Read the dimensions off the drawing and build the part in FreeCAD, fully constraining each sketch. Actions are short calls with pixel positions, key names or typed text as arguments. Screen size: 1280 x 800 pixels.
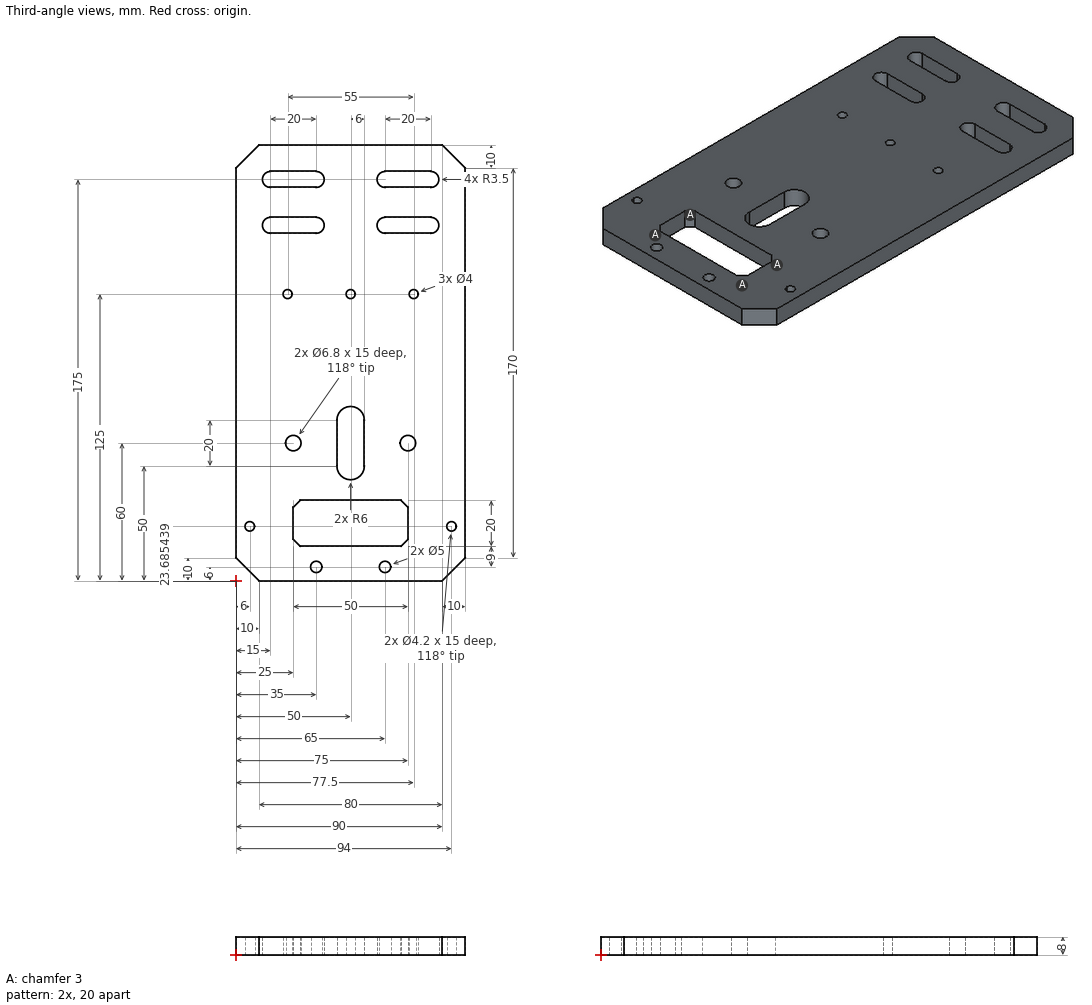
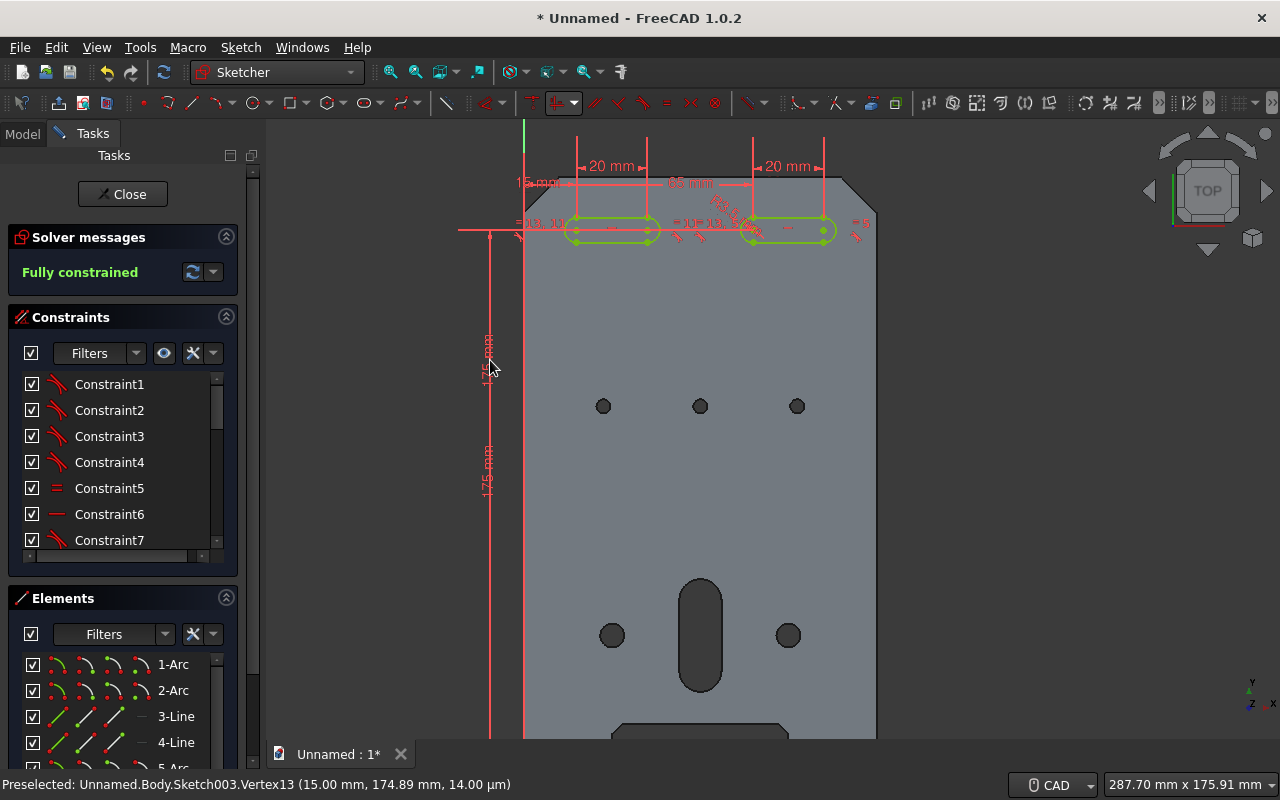
click(123, 194)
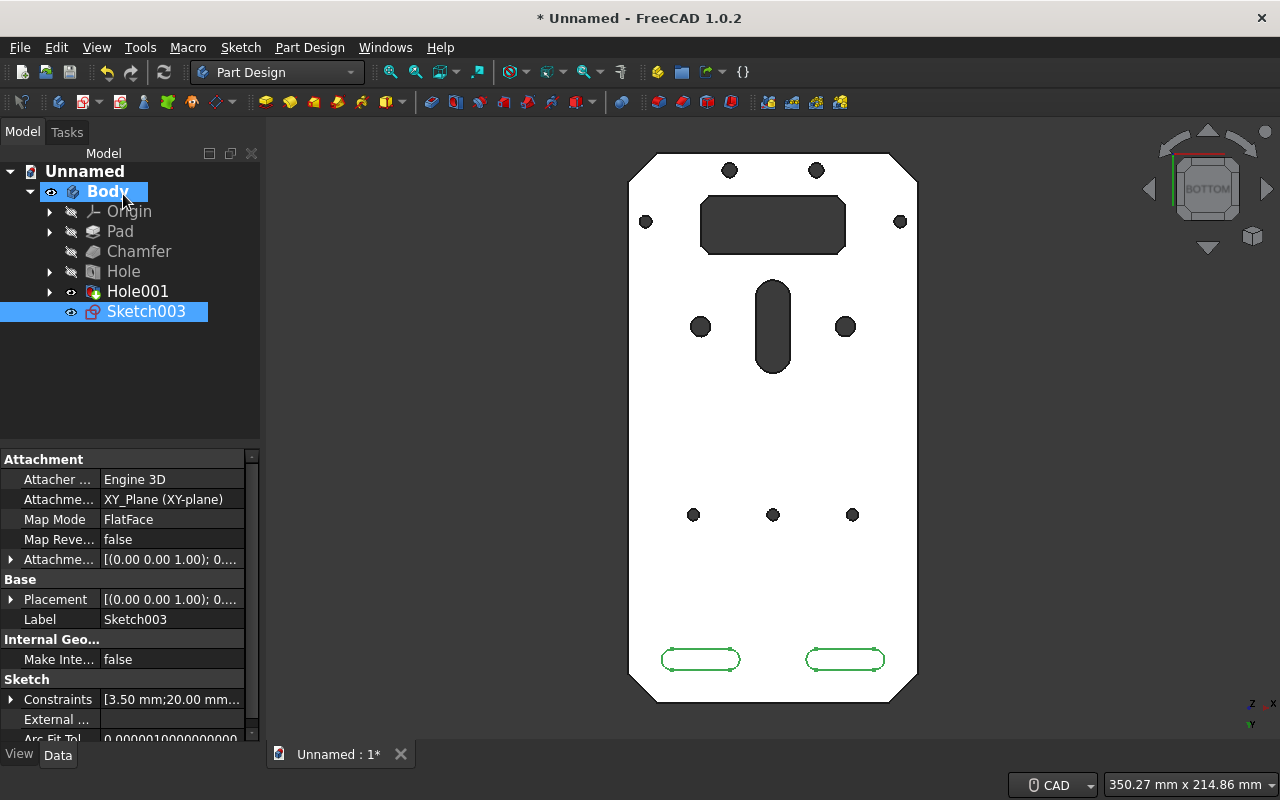
click(432, 102)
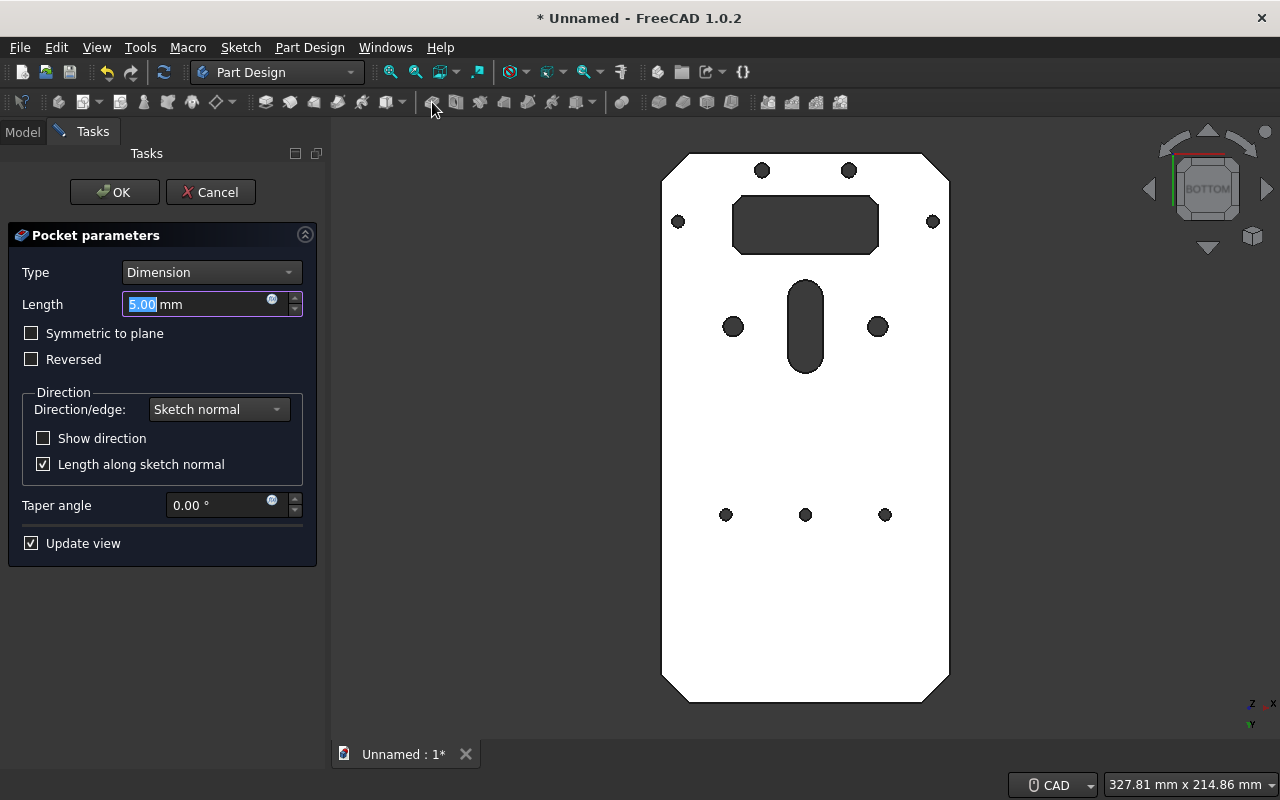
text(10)
key(Tab)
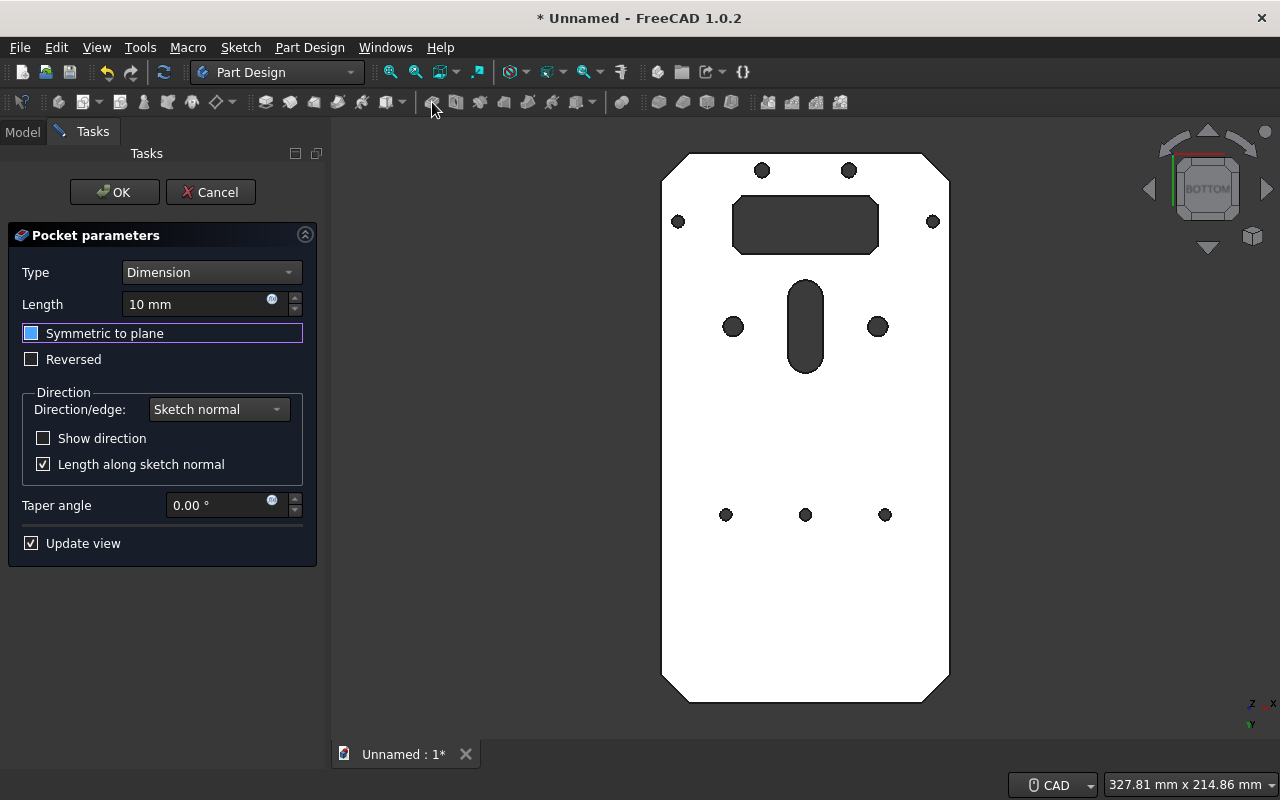
click(30, 359)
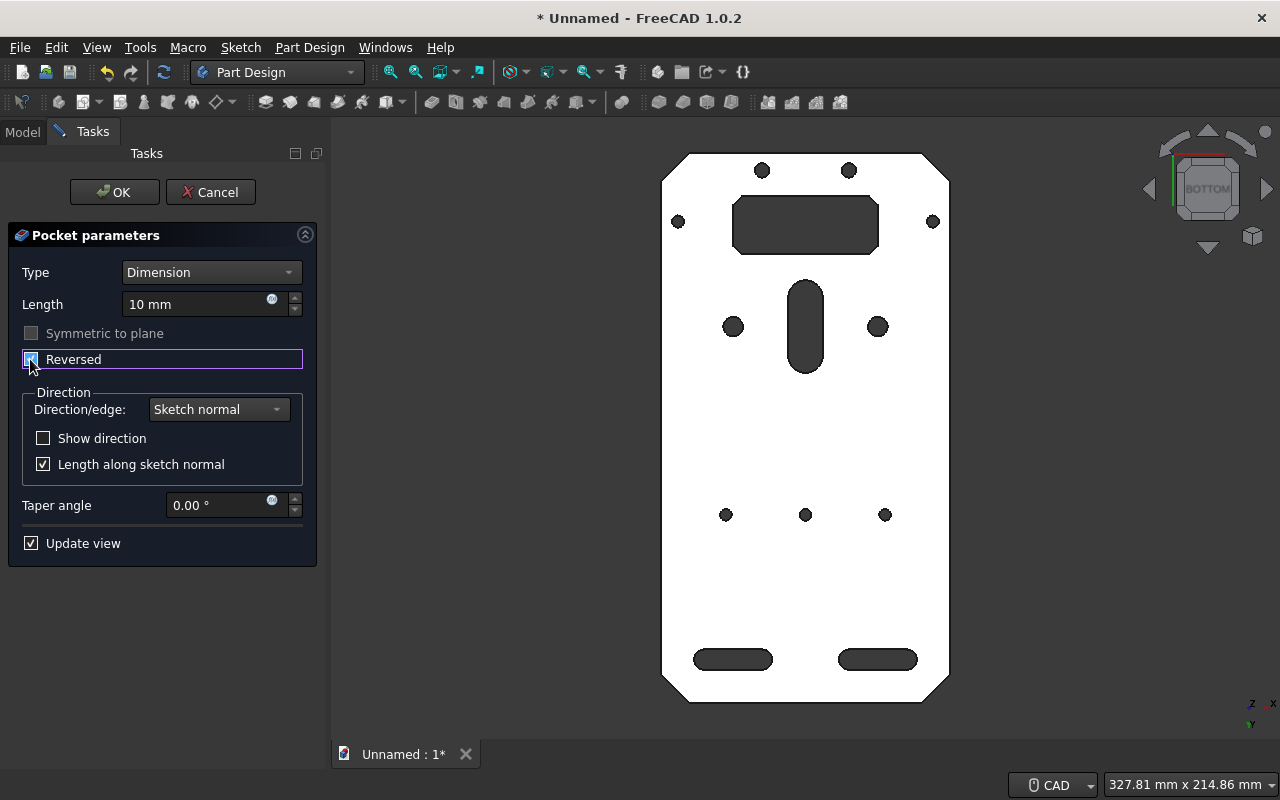
click(115, 192)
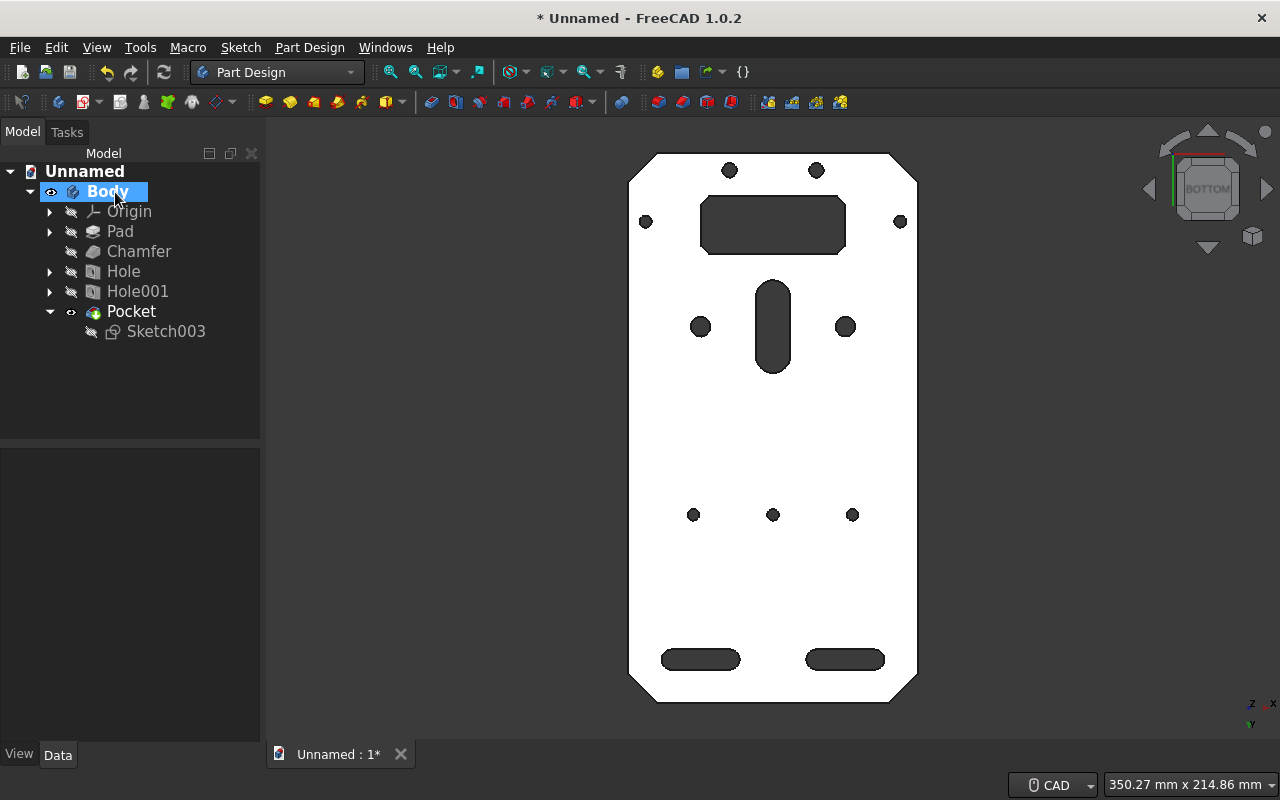
click(116, 312)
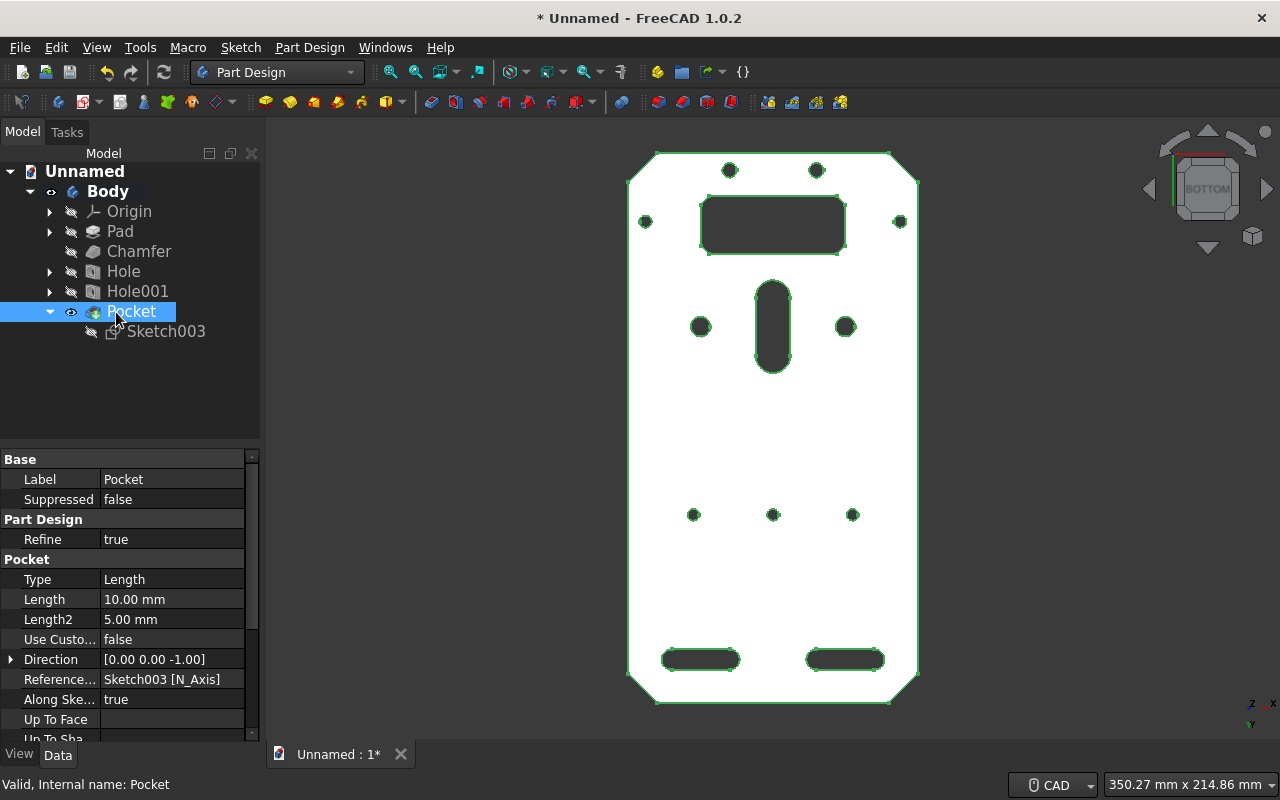
click(792, 102)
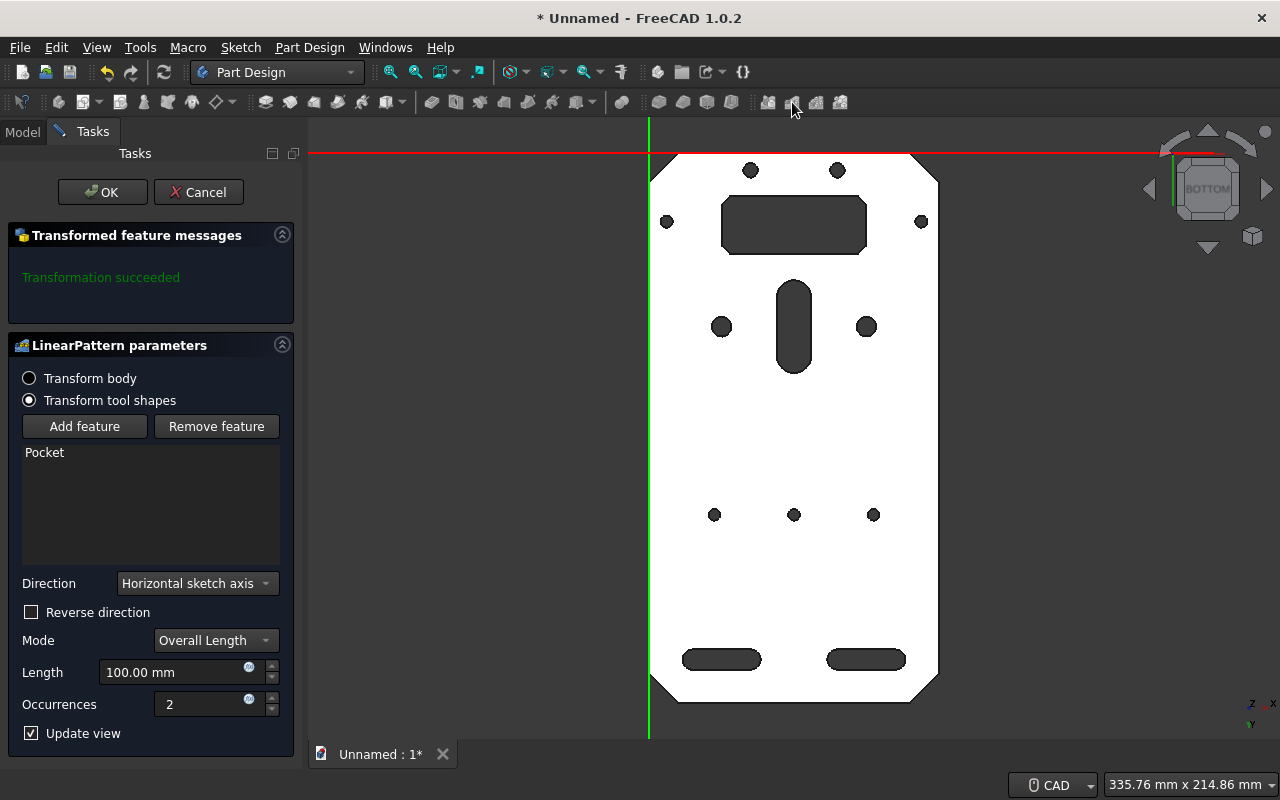
click(198, 584)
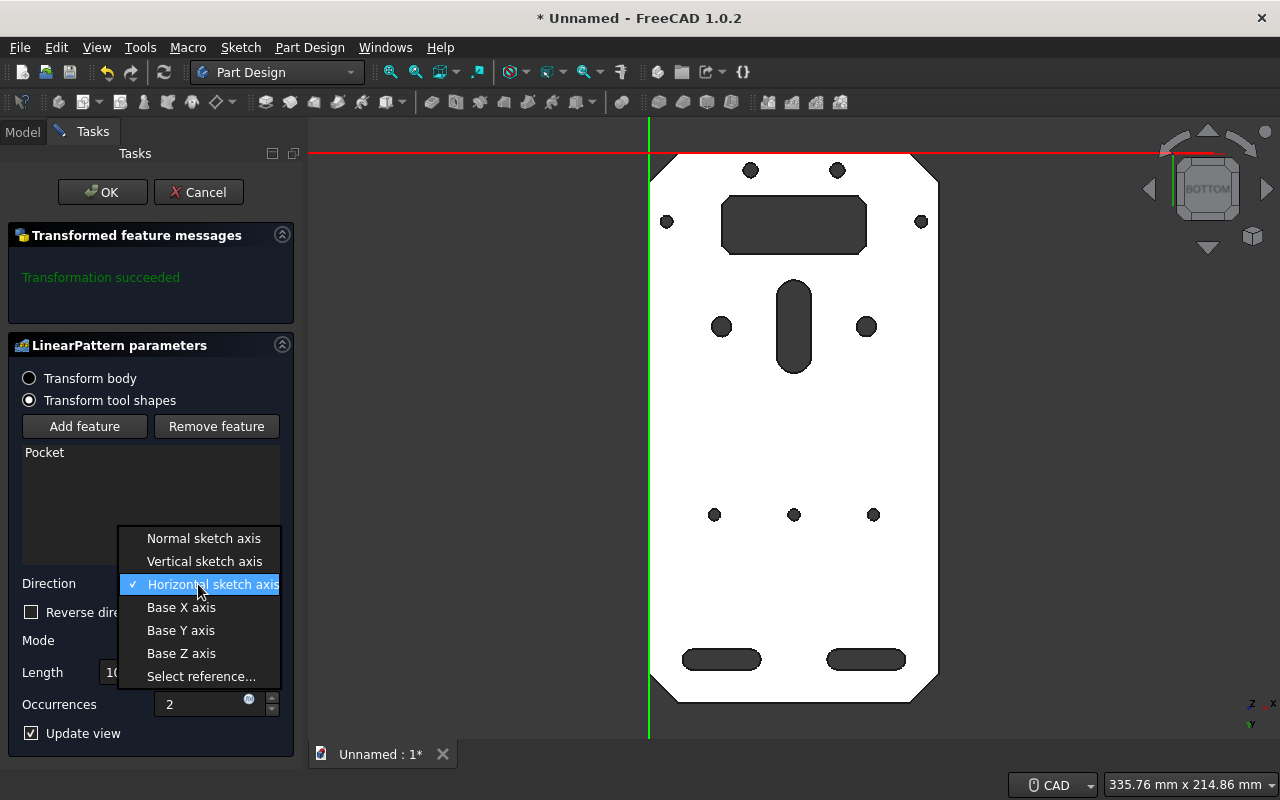
click(198, 630)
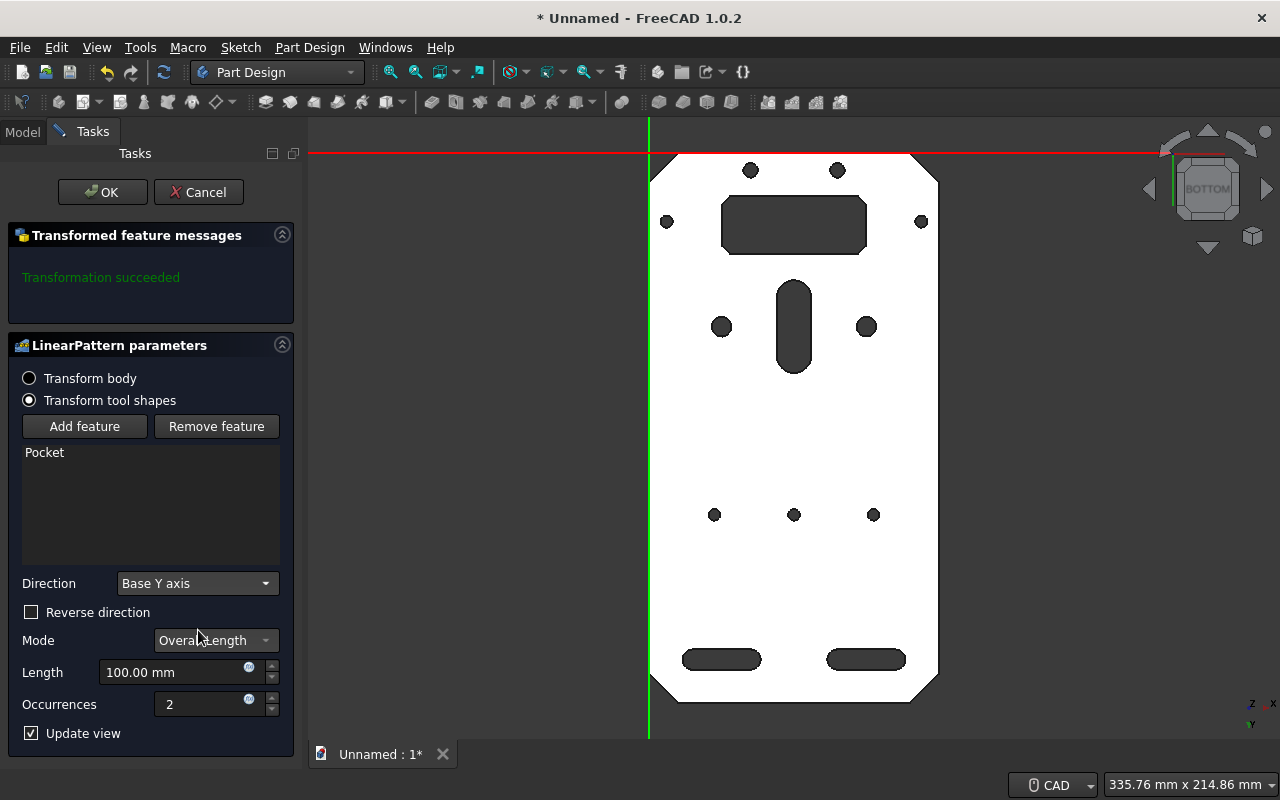
click(217, 640)